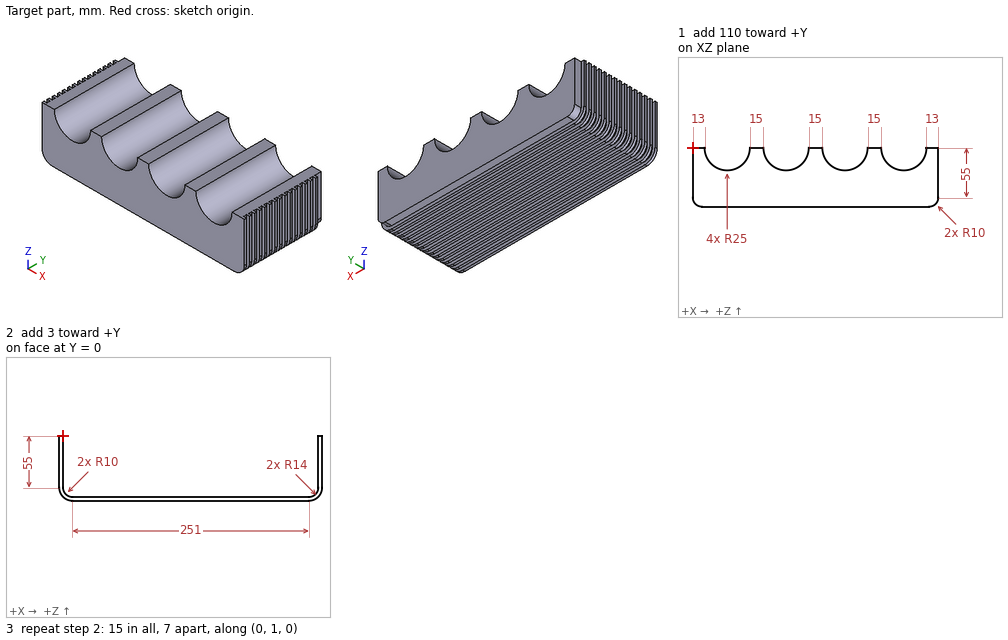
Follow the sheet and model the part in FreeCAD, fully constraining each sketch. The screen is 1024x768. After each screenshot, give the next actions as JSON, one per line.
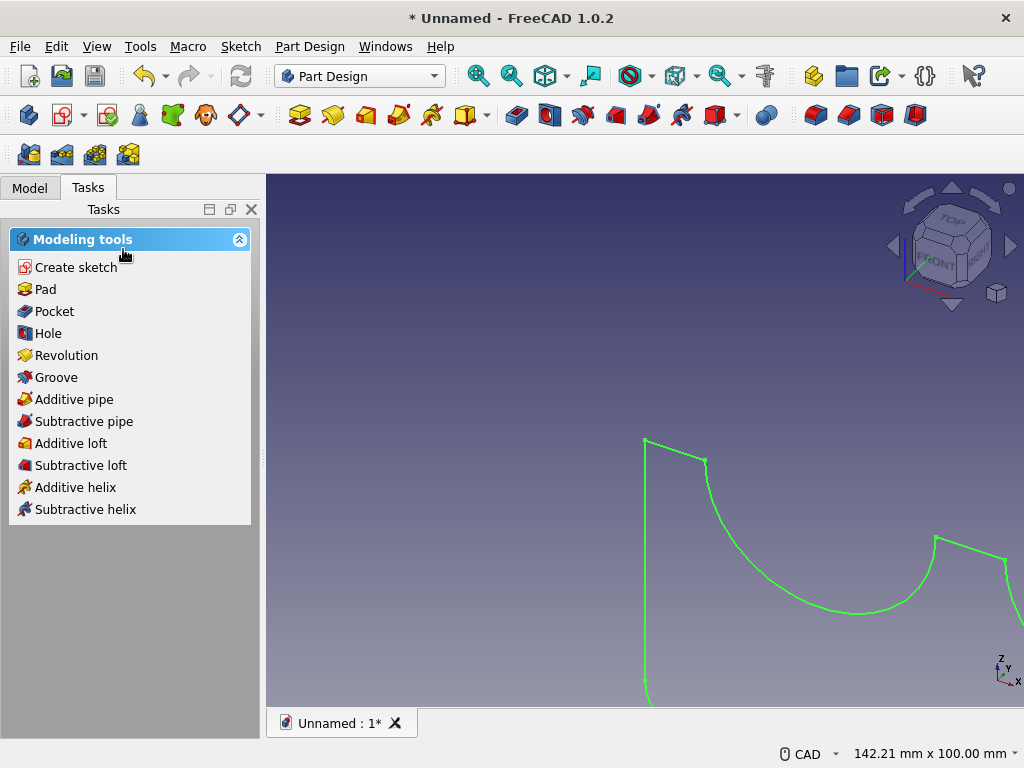
{"action": "left_click", "coordinate": [300, 116]}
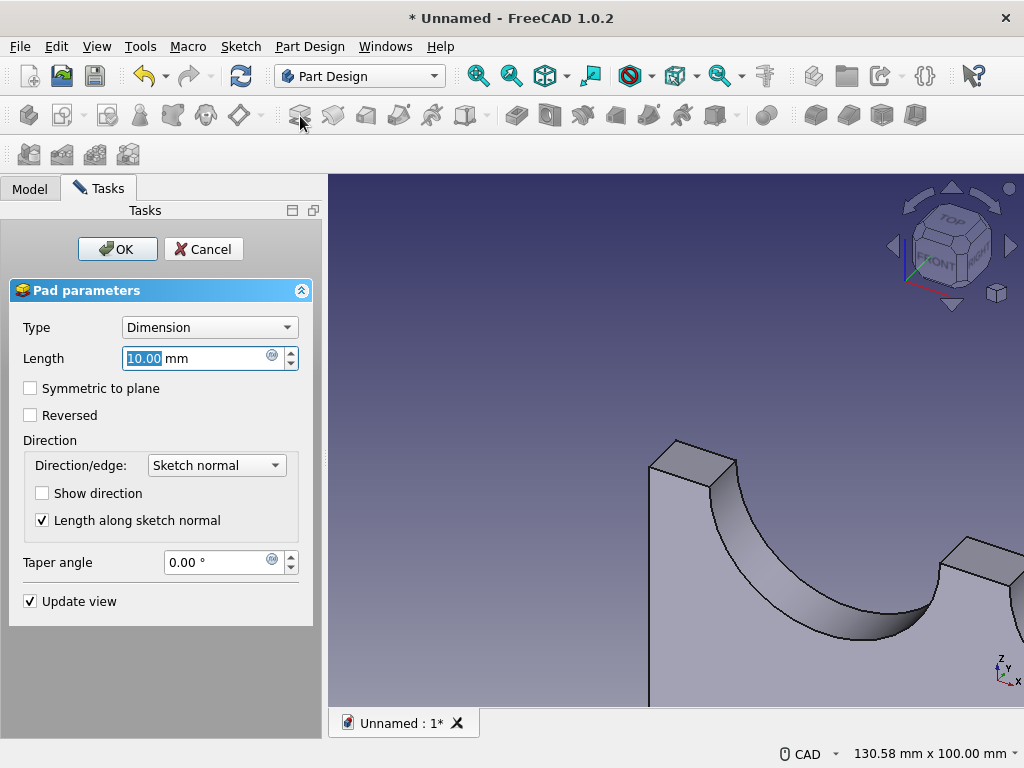
{"action": "type", "text": "110"}
{"action": "key", "text": "Tab"}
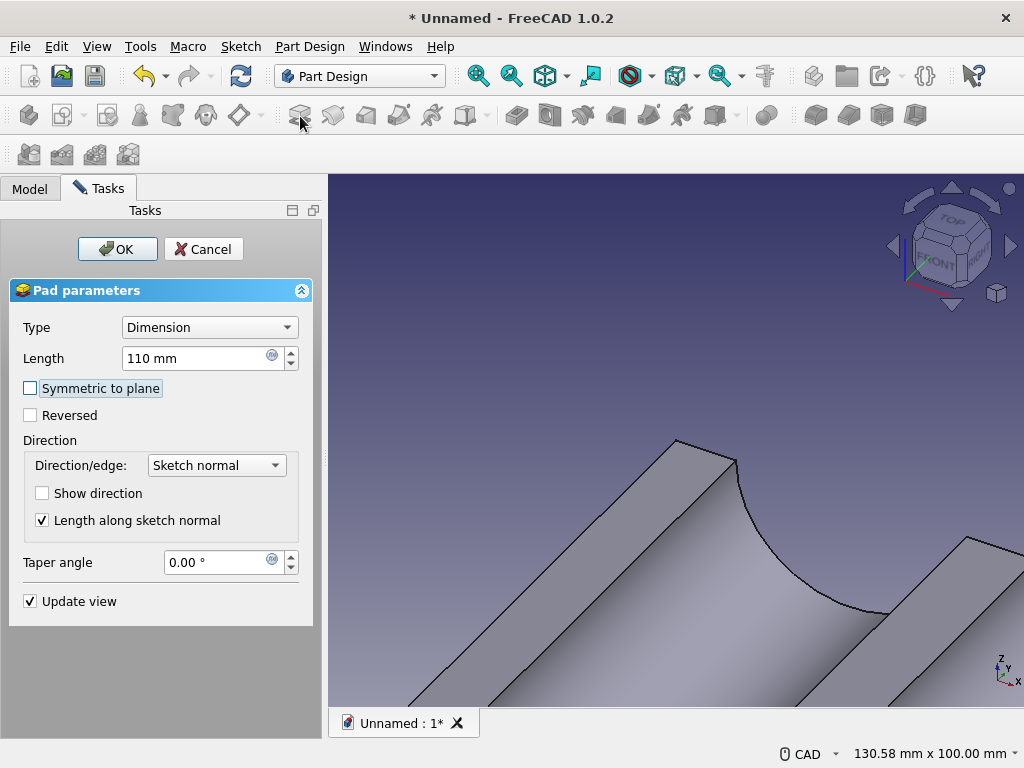
{"action": "left_click", "coordinate": [31, 415]}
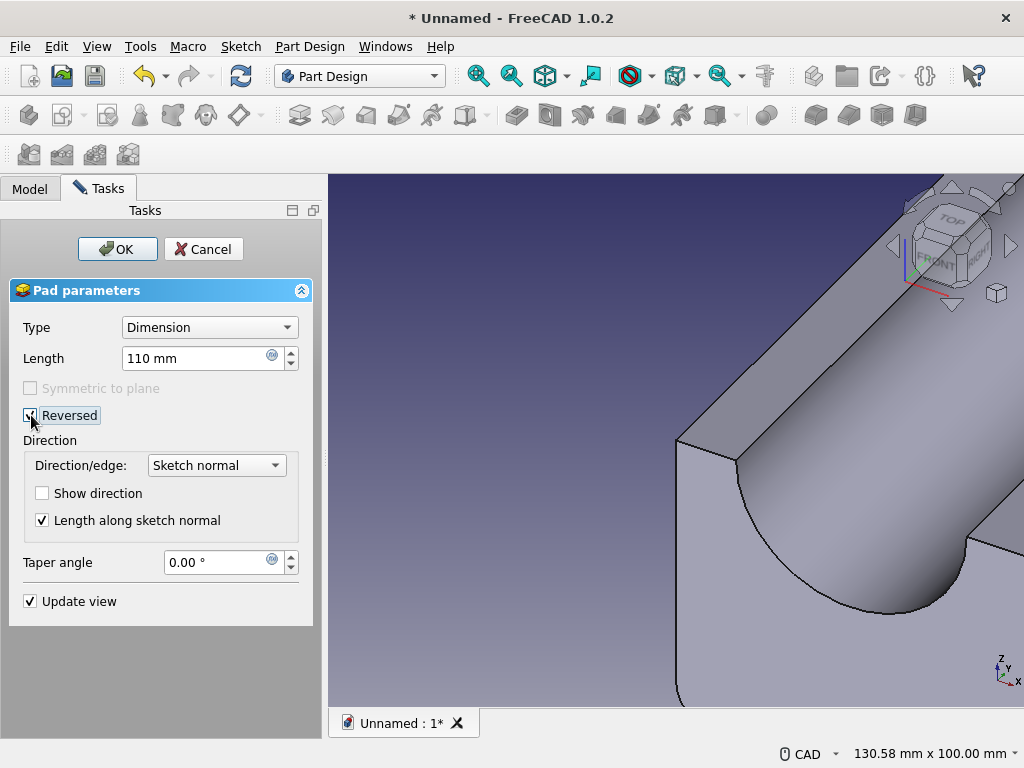
{"action": "left_click", "coordinate": [118, 249]}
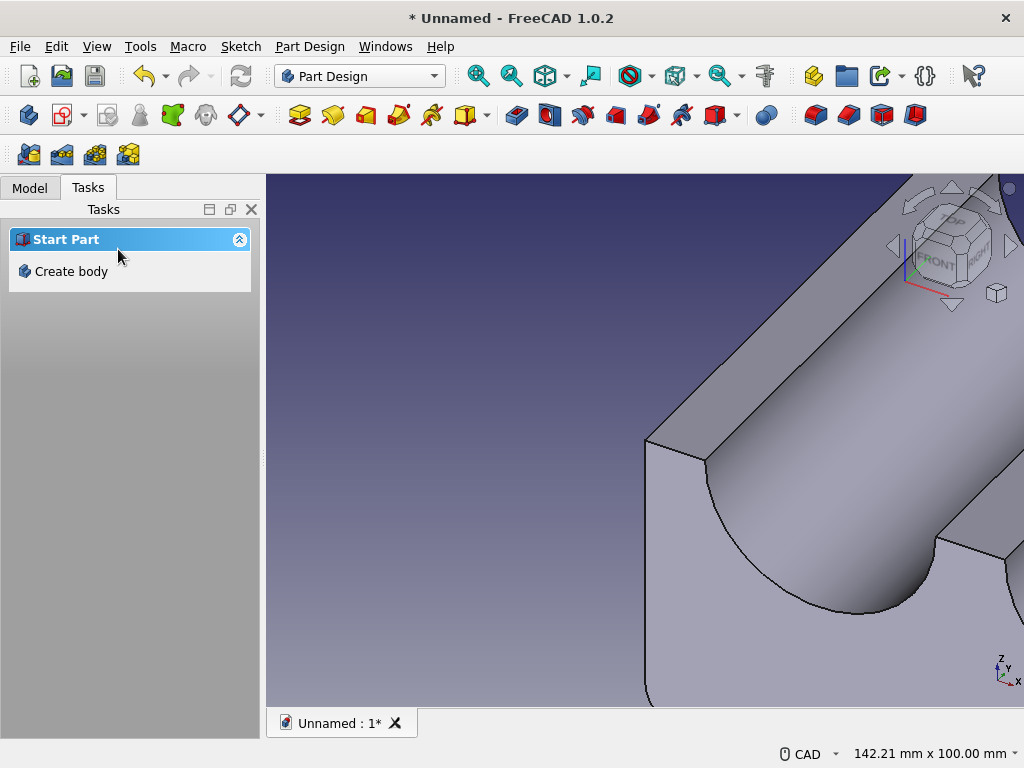
{"action": "left_click", "coordinate": [479, 76]}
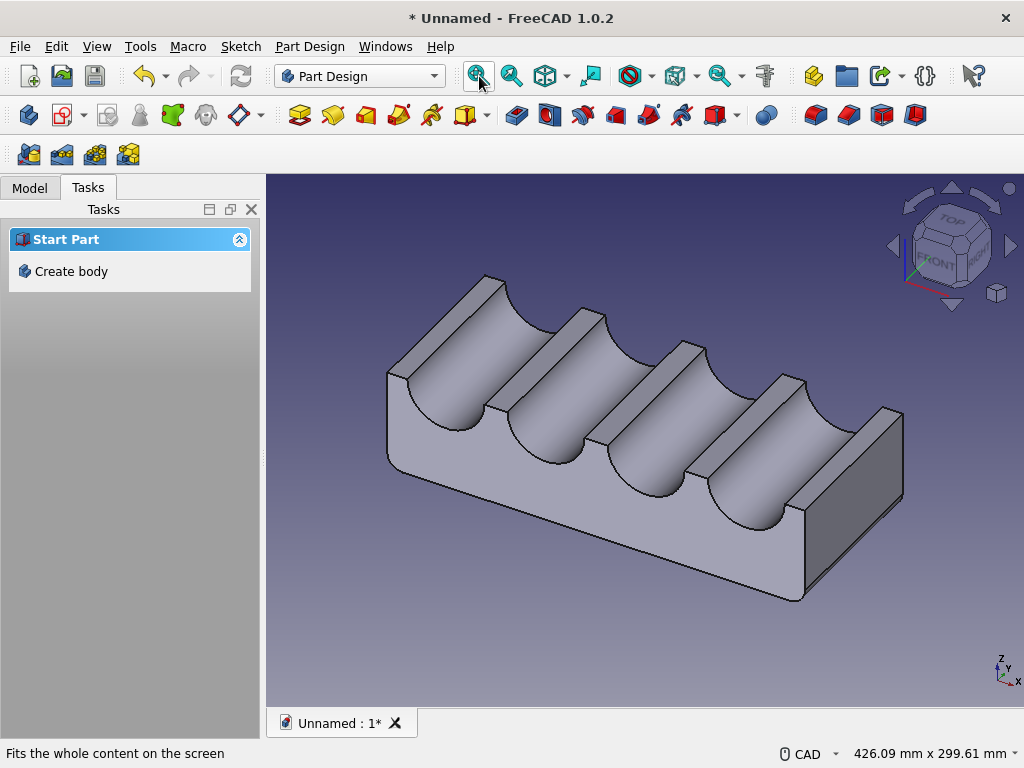
{"action": "left_click", "coordinate": [596, 502]}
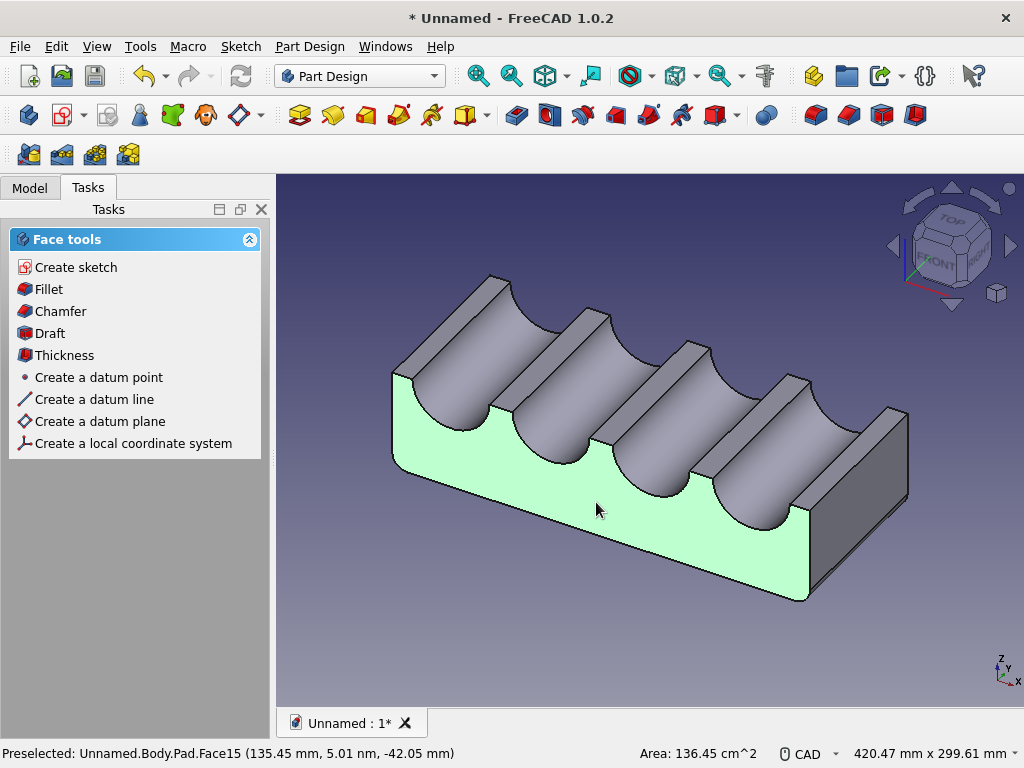
{"action": "left_click", "coordinate": [62, 116]}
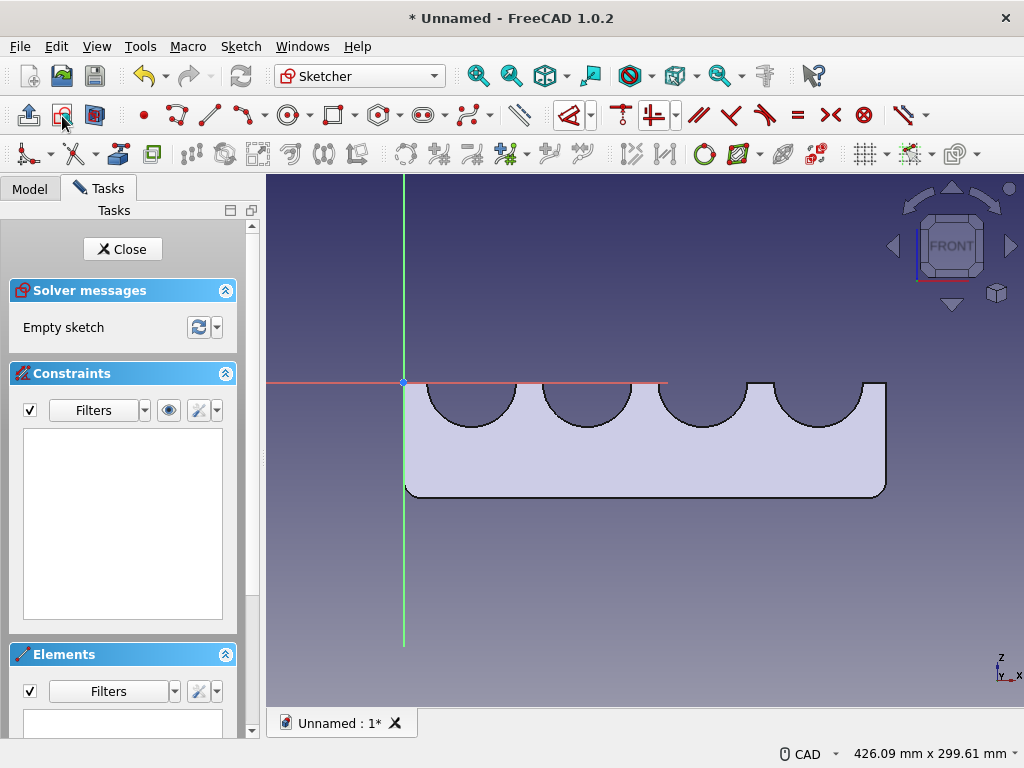
{"action": "scroll", "coordinate": [294, 424], "scroll_direction": "down", "scroll_amount": 1}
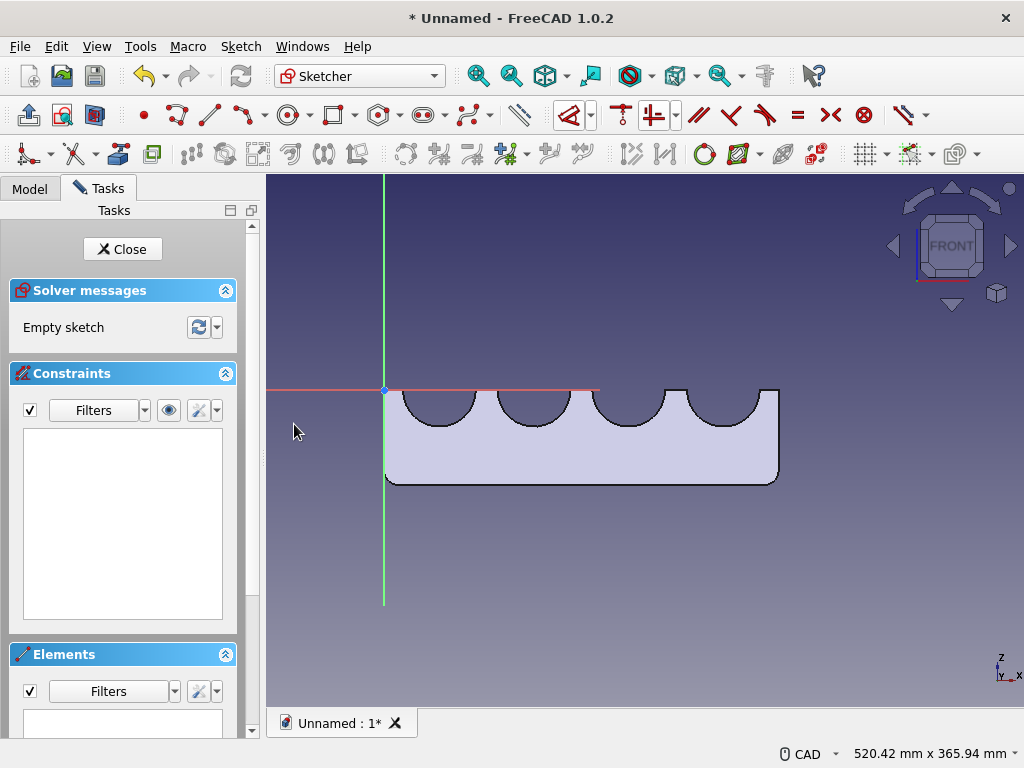
{"action": "left_click", "coordinate": [210, 116]}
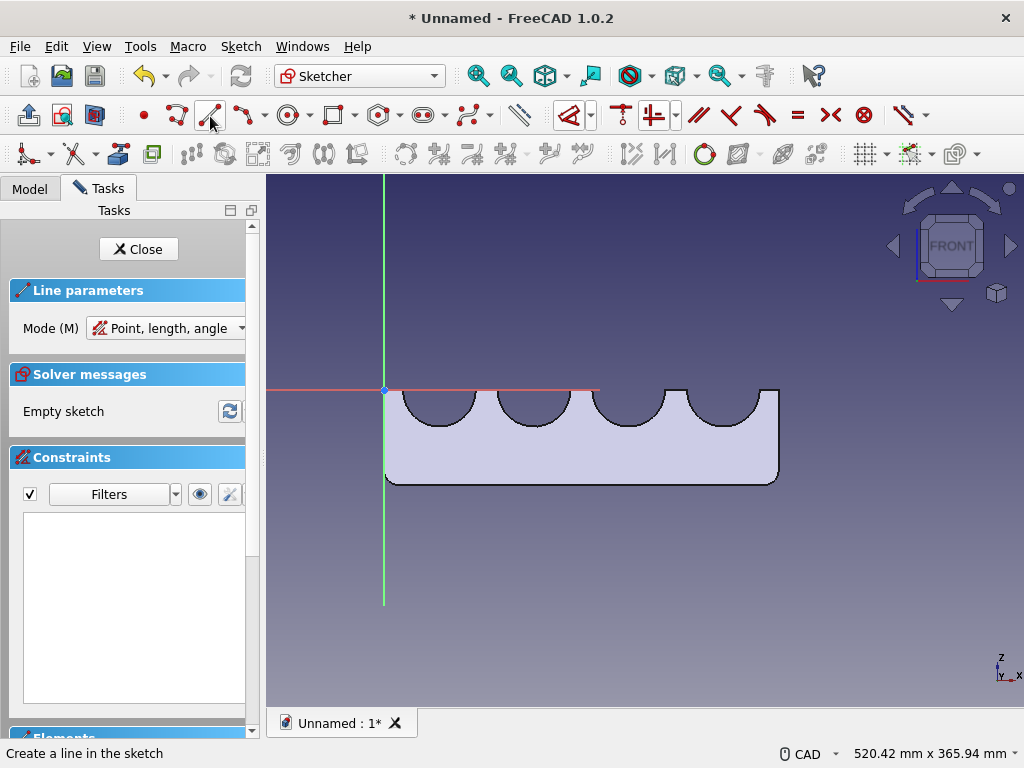
{"action": "left_click", "coordinate": [764, 491]}
{"action": "left_click", "coordinate": [399, 491]}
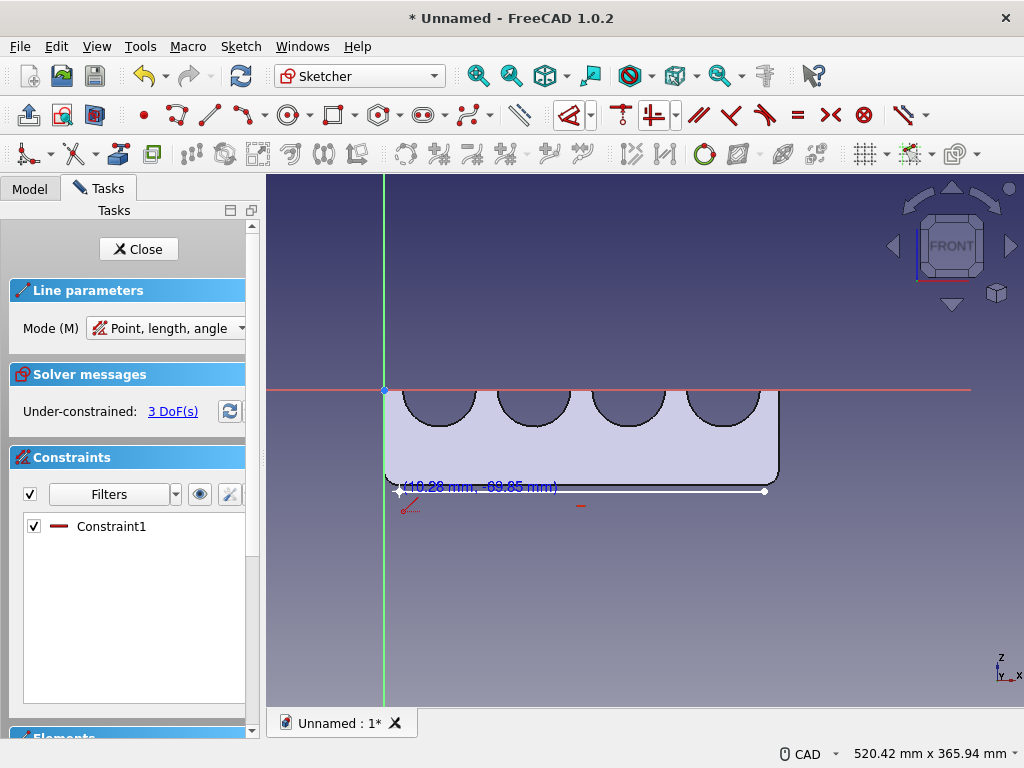
{"action": "left_click", "coordinate": [177, 116]}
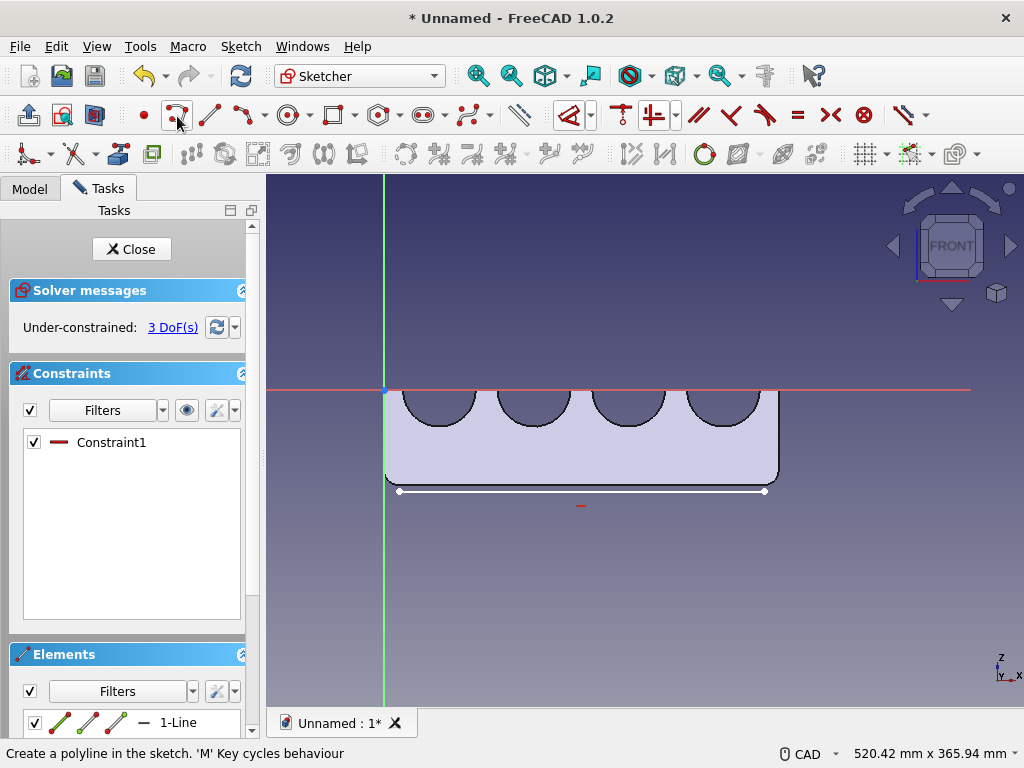
{"action": "scroll", "coordinate": [378, 470], "scroll_direction": "up", "scroll_amount": 6}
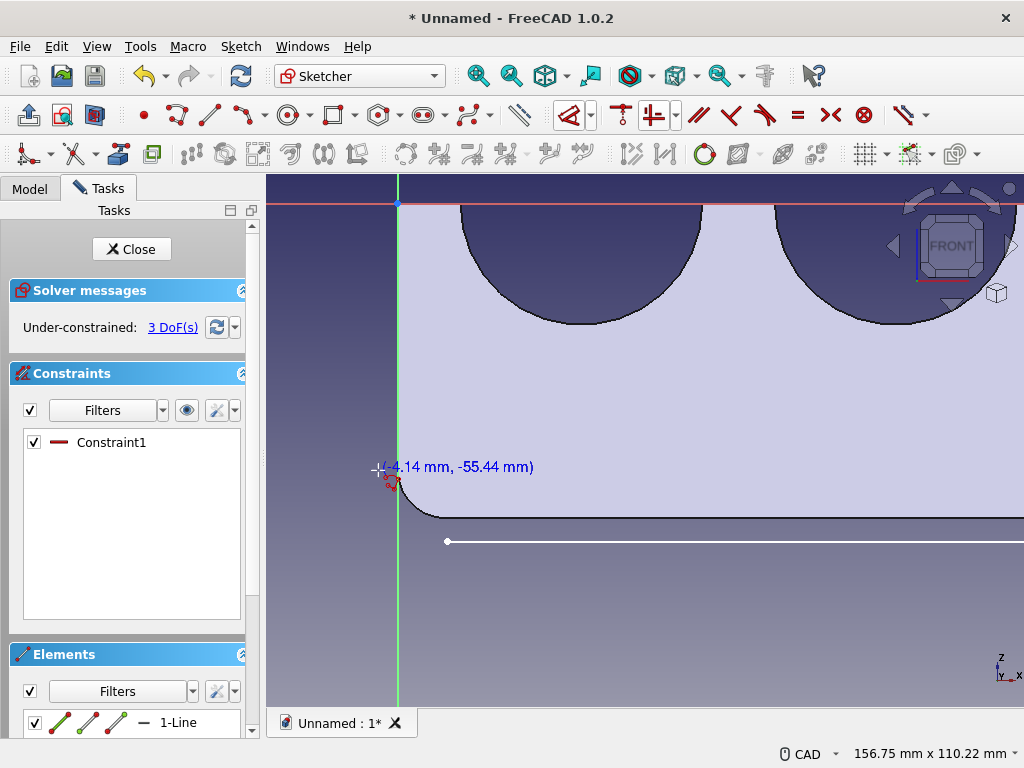
{"action": "left_click", "coordinate": [378, 470]}
{"action": "left_click", "coordinate": [378, 204]}
{"action": "left_click", "coordinate": [398, 204]}
{"action": "left_click", "coordinate": [407, 470]}
{"action": "right_click", "coordinate": [407, 470]}